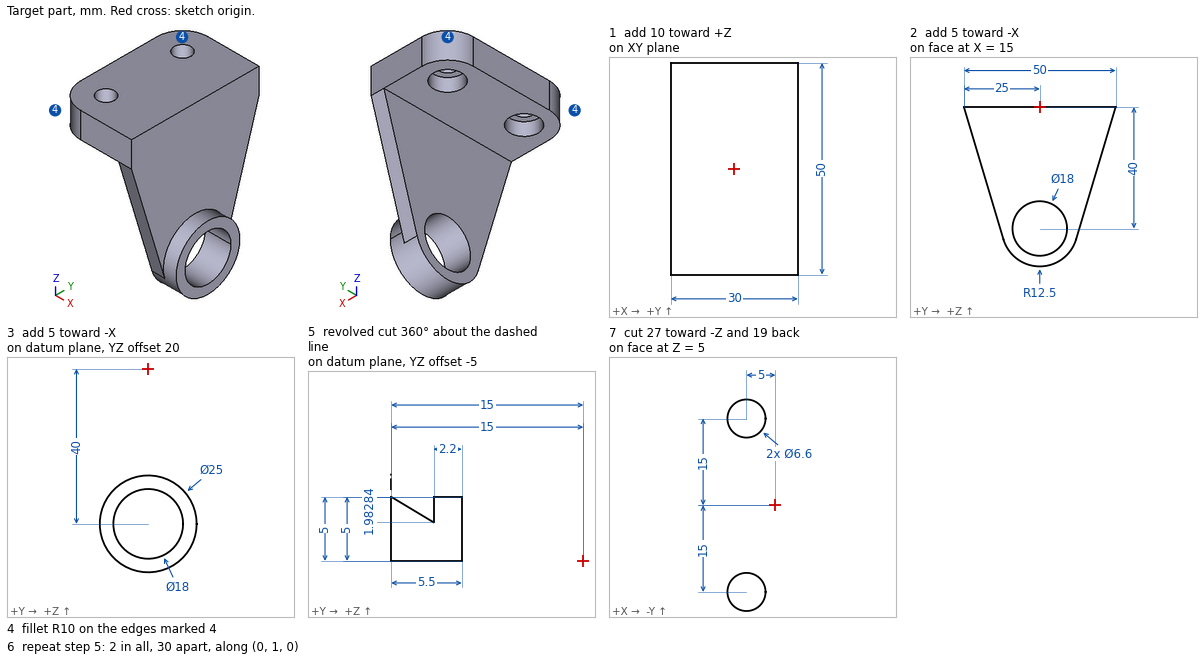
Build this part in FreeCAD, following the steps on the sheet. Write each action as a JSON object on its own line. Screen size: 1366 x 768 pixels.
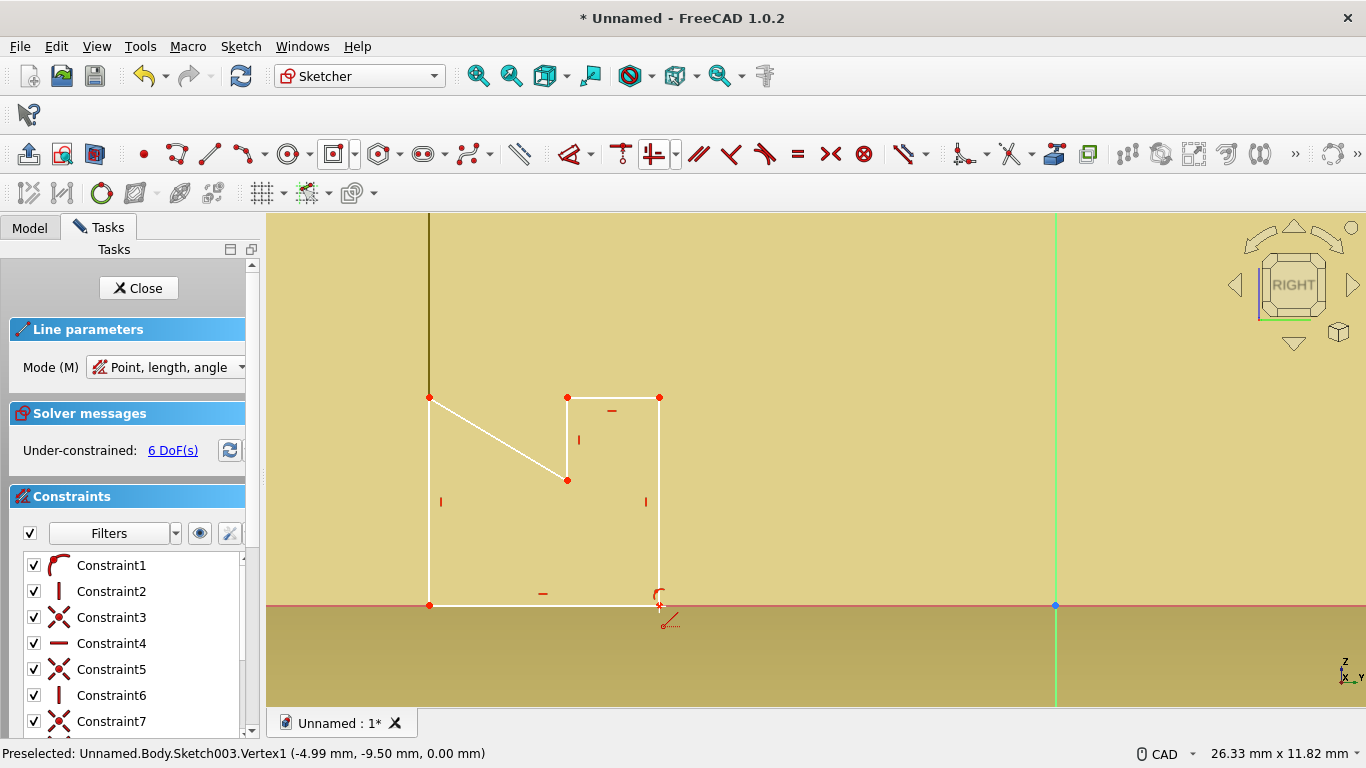
{"action": "left_click", "coordinate": [429, 376]}
{"action": "left_click", "coordinate": [429, 314]}
{"action": "key", "text": "Escape"}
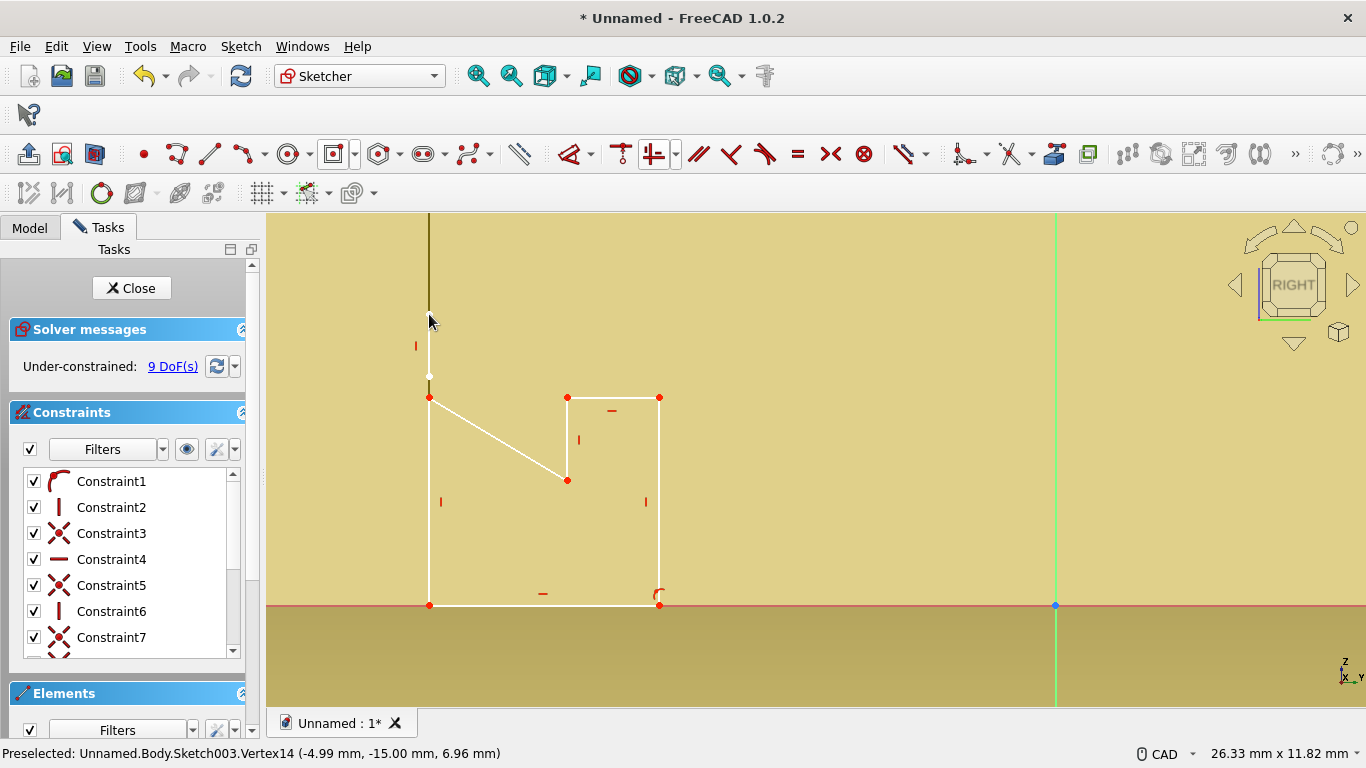
{"action": "left_click", "coordinate": [429, 358]}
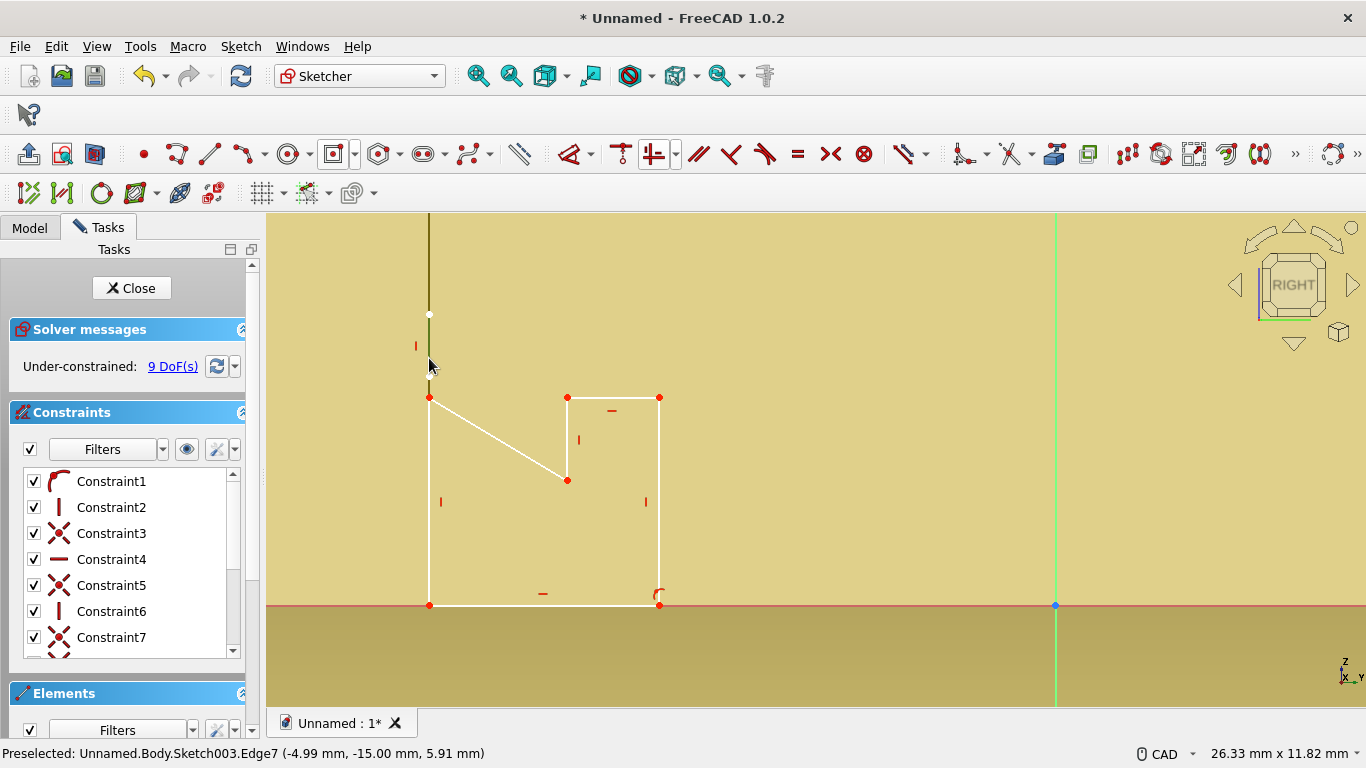
{"action": "left_click", "coordinate": [520, 154]}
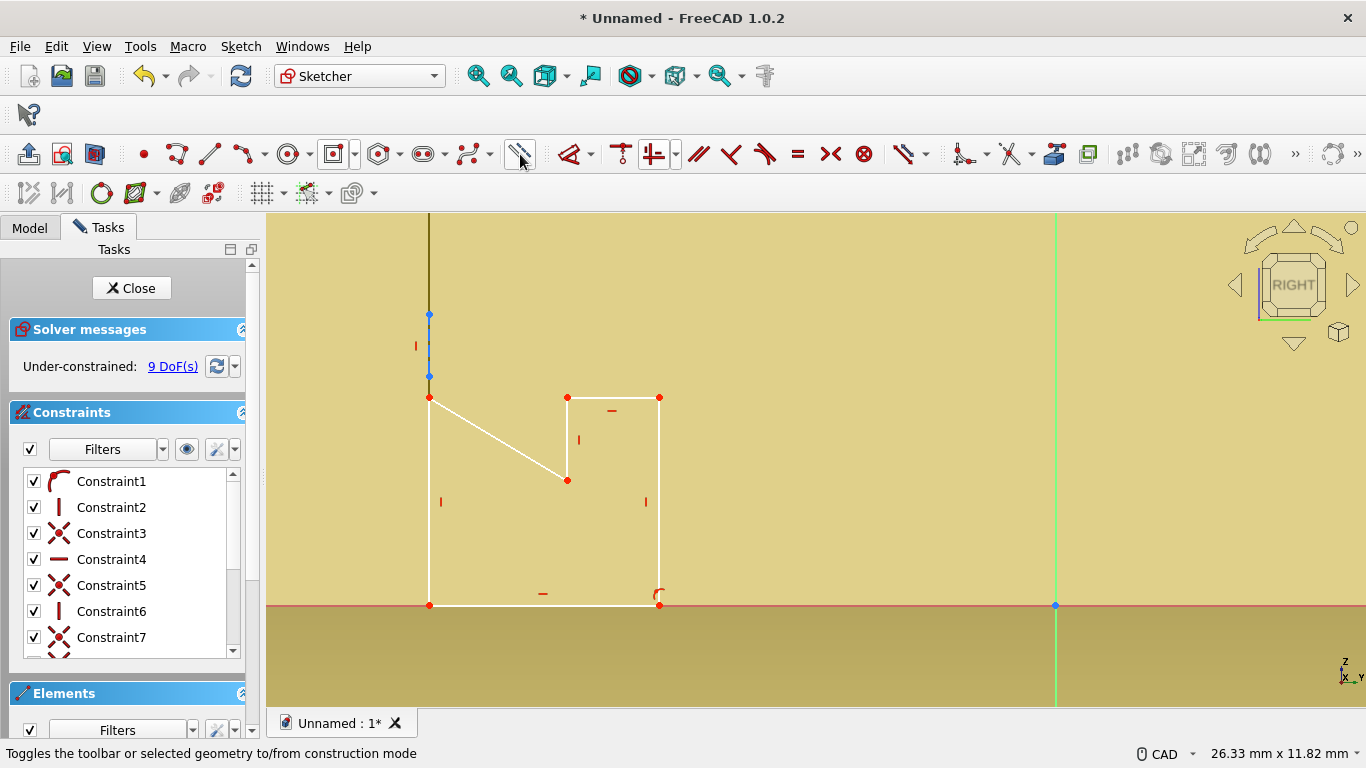
{"action": "left_click", "coordinate": [568, 154]}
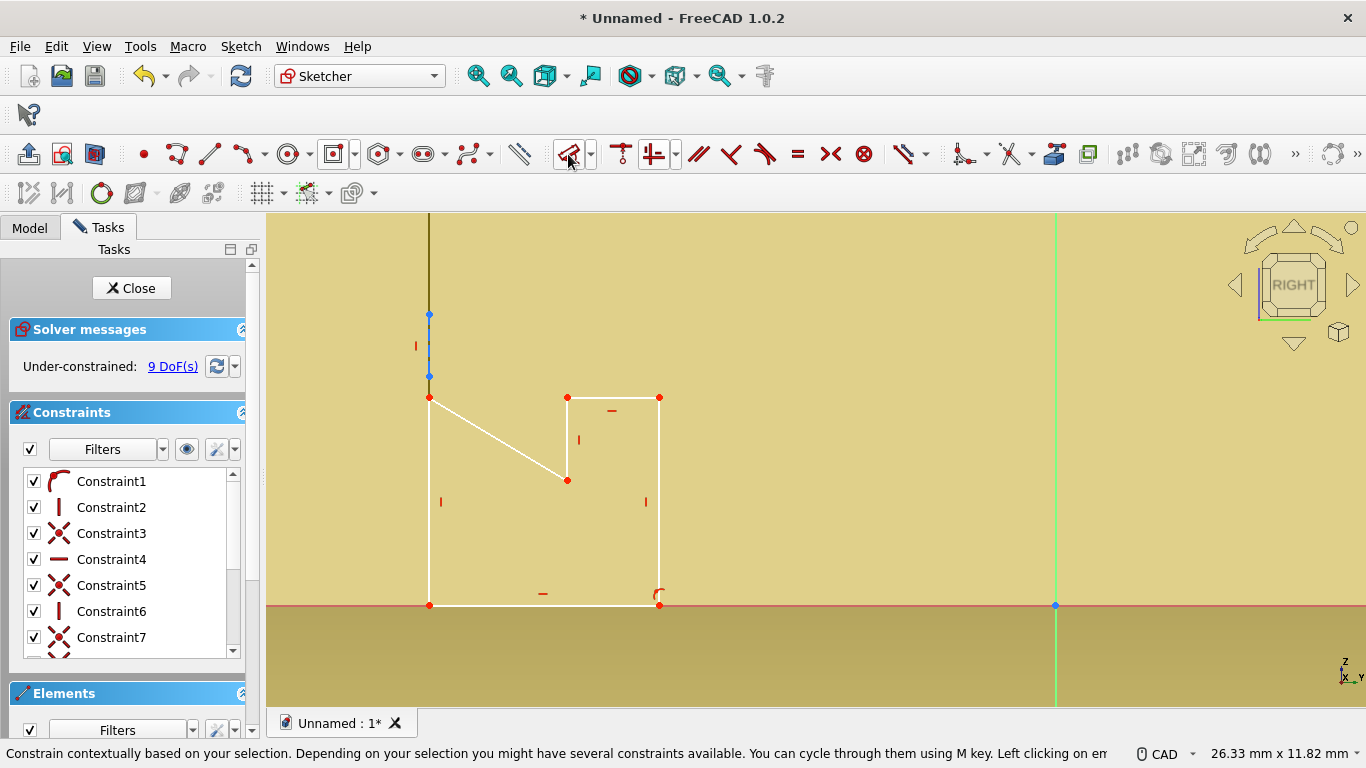
{"action": "left_click", "coordinate": [659, 544]}
{"action": "left_click", "coordinate": [625, 502]}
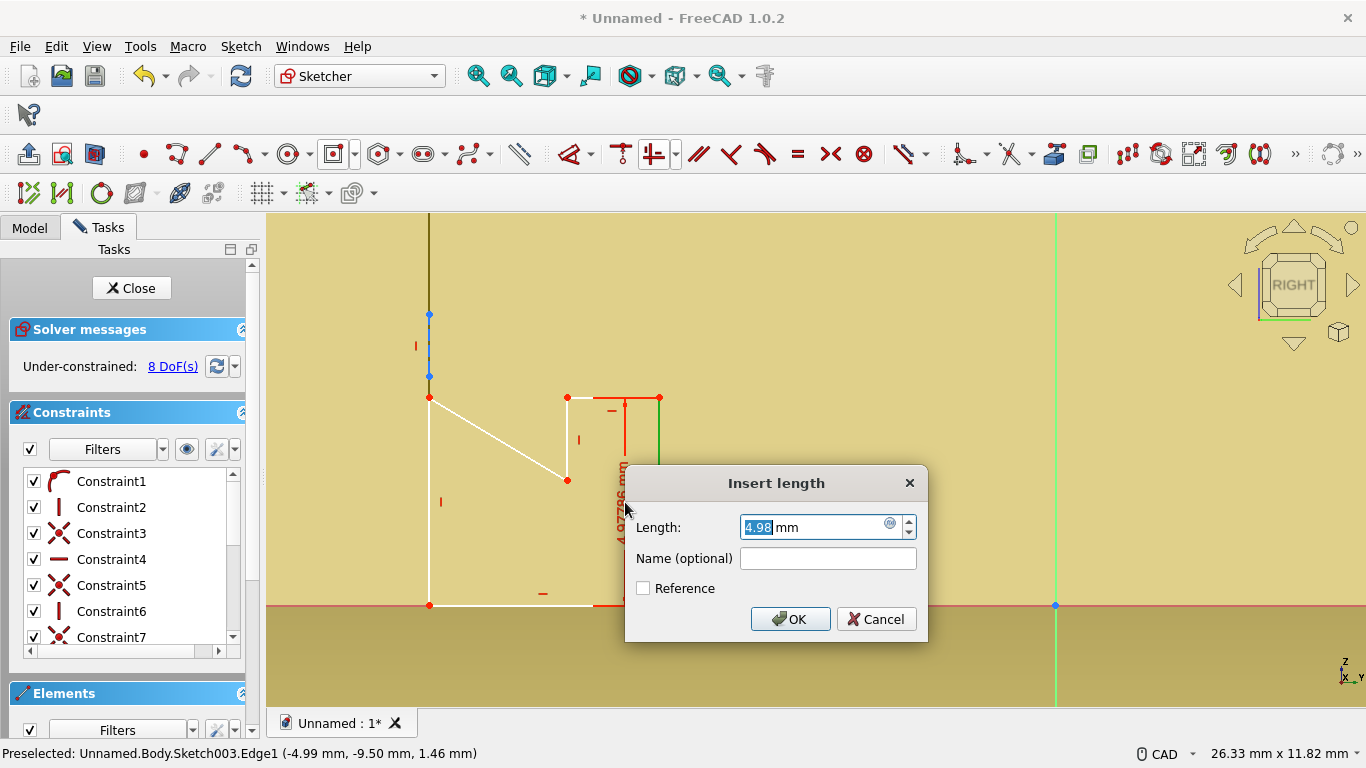
{"action": "type", "text": "5"}
{"action": "key", "text": "Return"}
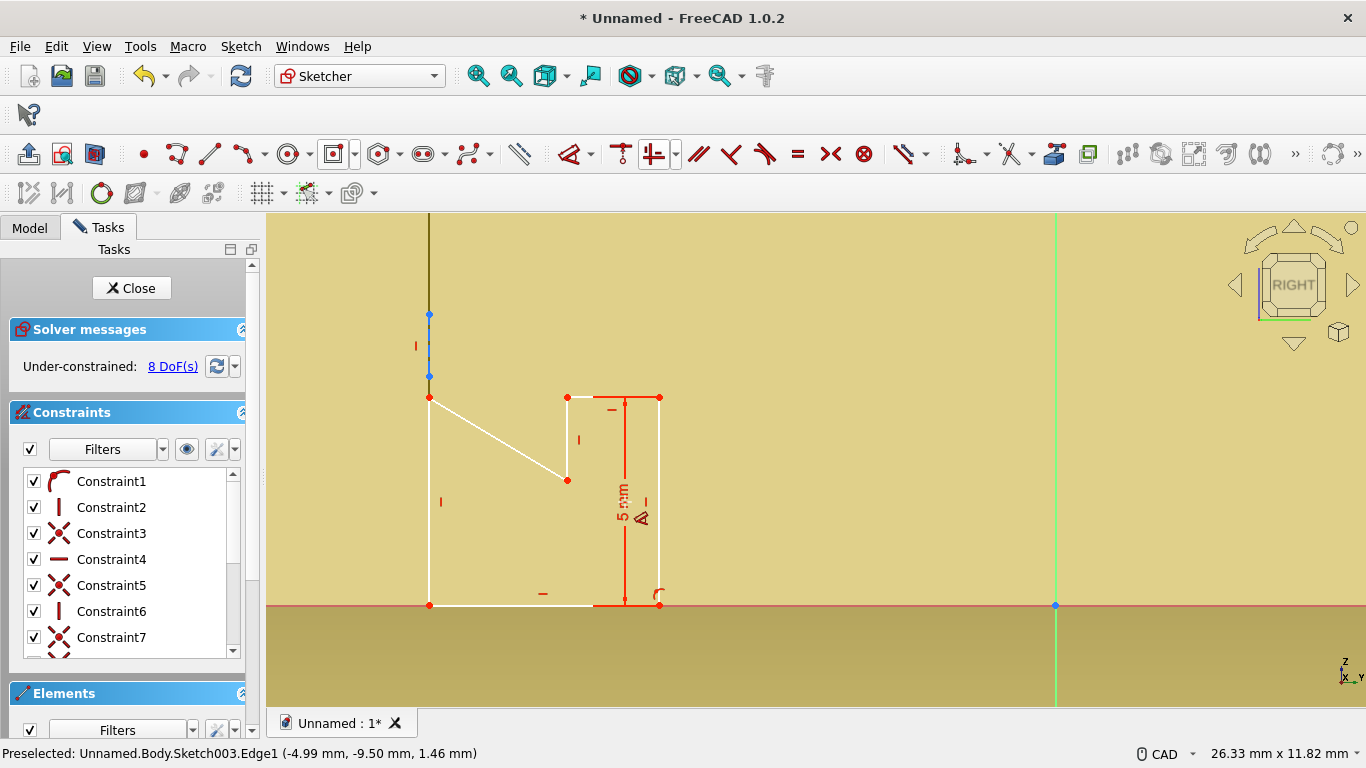
{"action": "left_click", "coordinate": [429, 460]}
{"action": "left_click", "coordinate": [395, 502]}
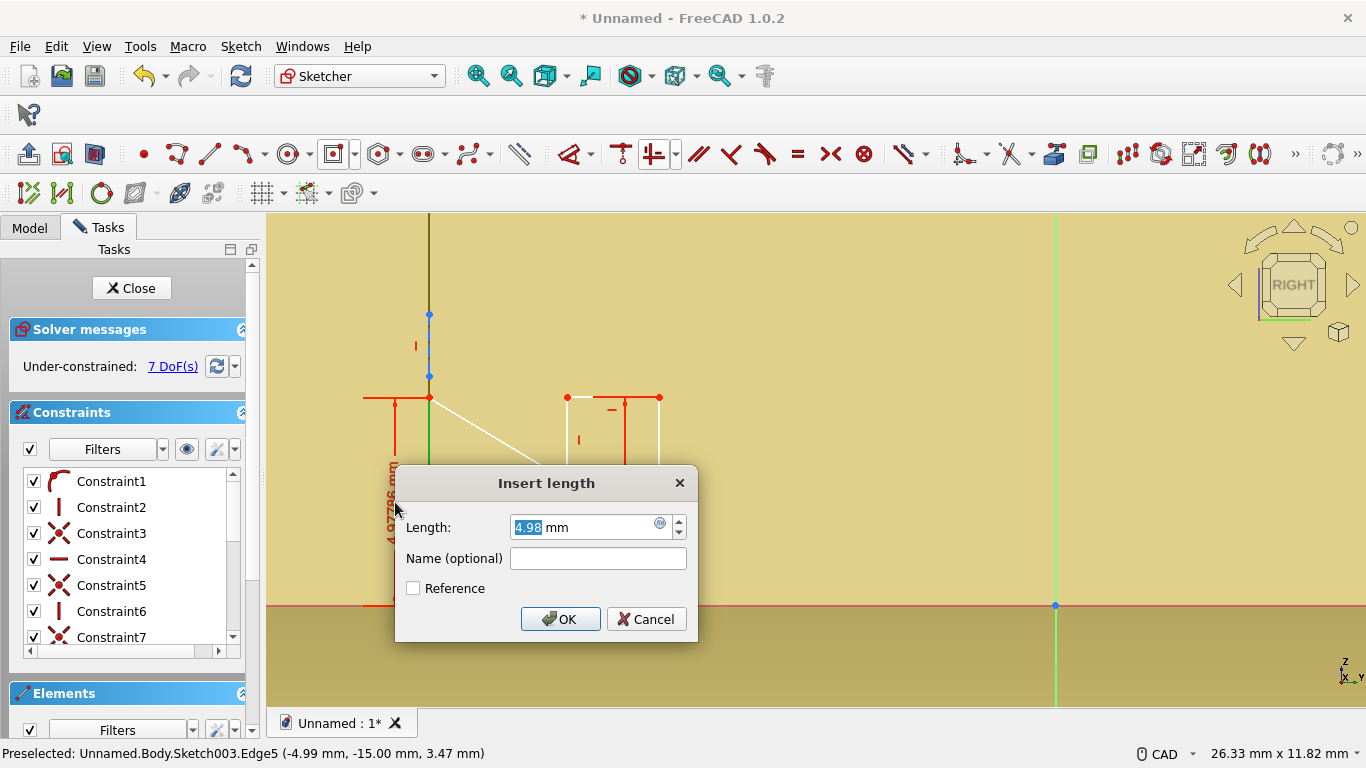
{"action": "type", "text": "5"}
{"action": "key", "text": "Return"}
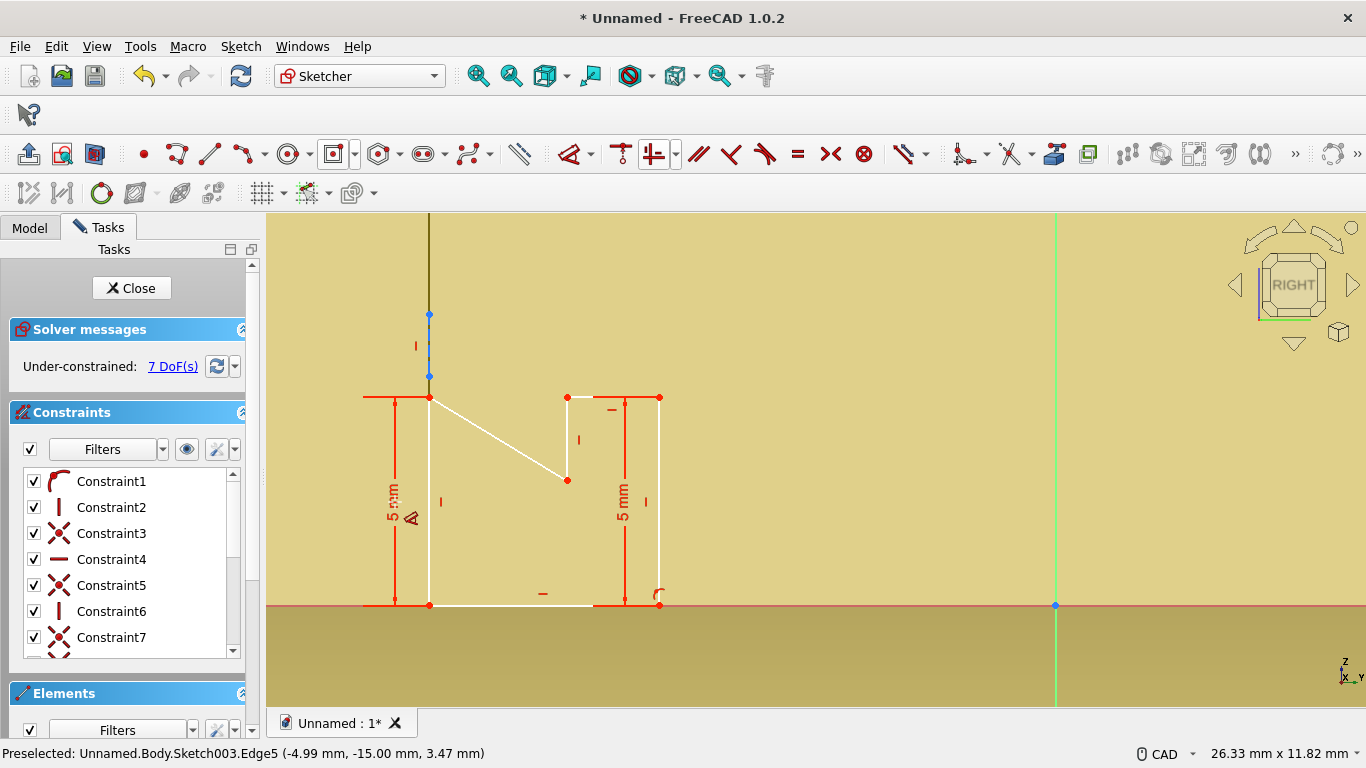
{"action": "left_click", "coordinate": [631, 397]}
{"action": "left_click", "coordinate": [613, 363]}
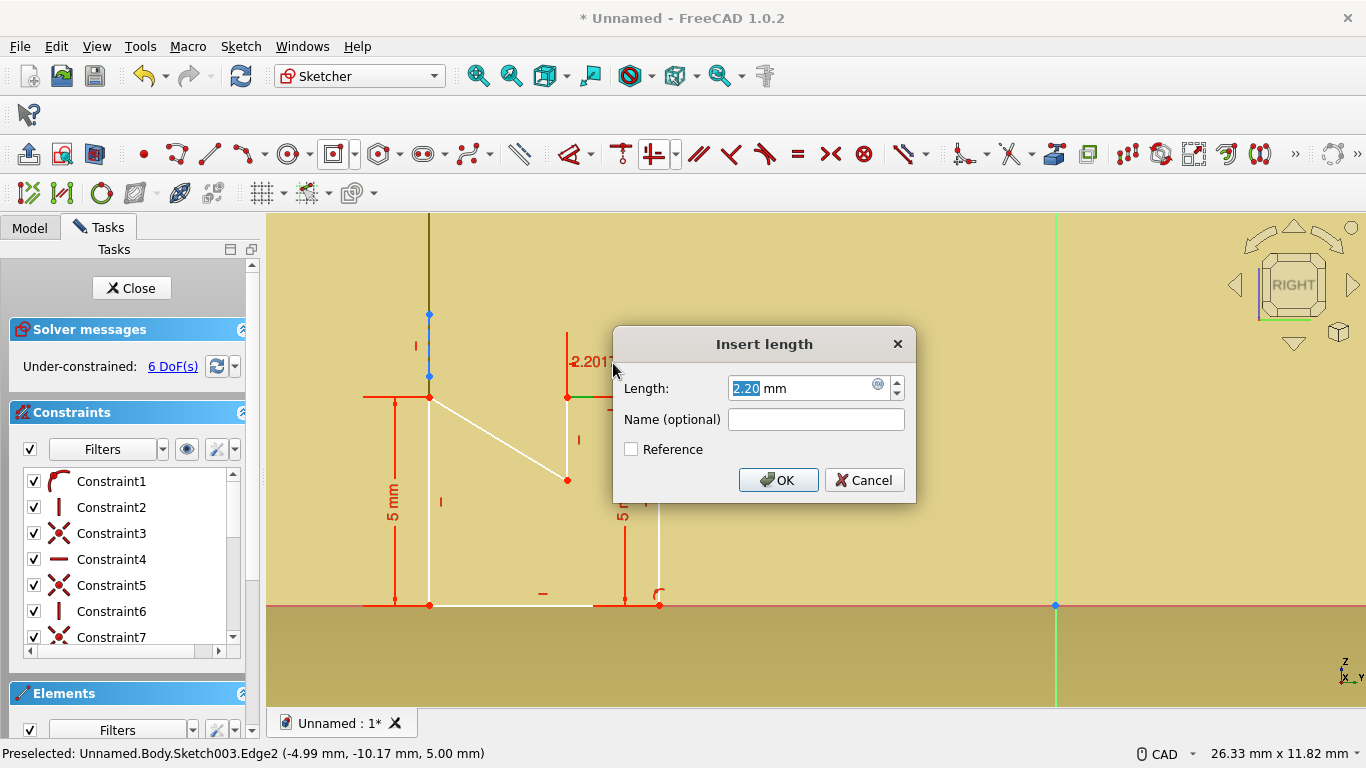
{"action": "type", "text": "2.2"}
{"action": "key", "text": "Return"}